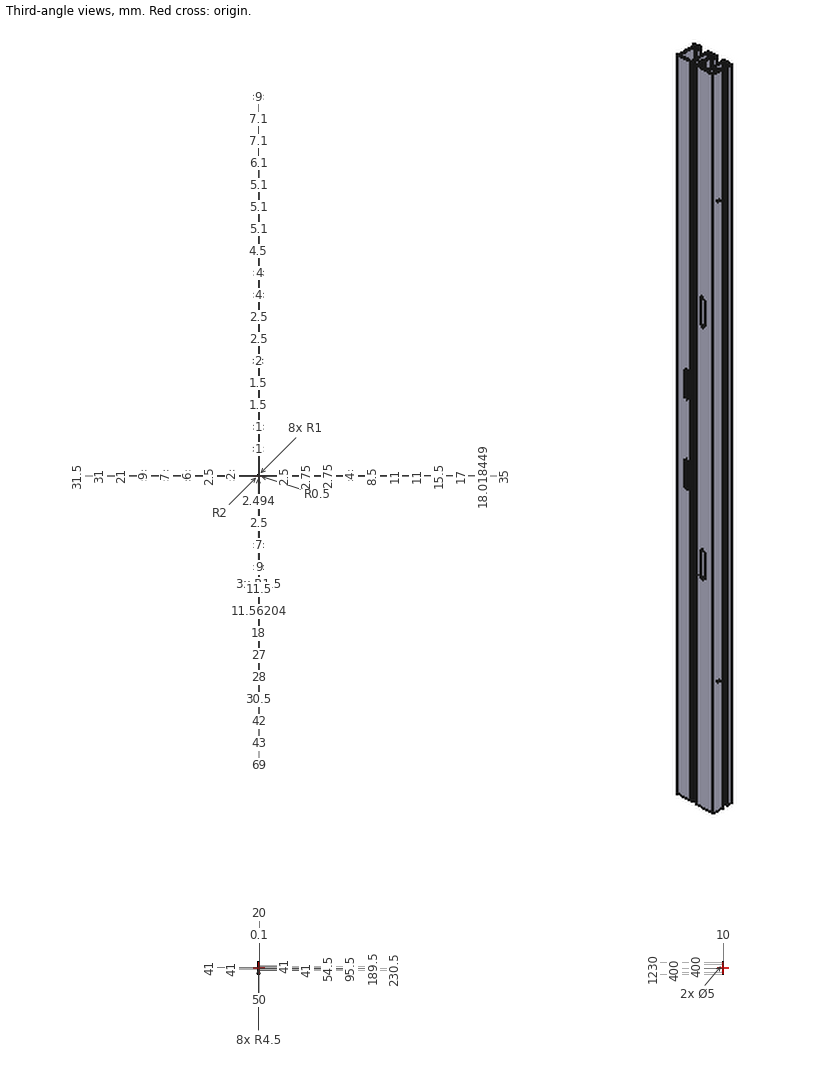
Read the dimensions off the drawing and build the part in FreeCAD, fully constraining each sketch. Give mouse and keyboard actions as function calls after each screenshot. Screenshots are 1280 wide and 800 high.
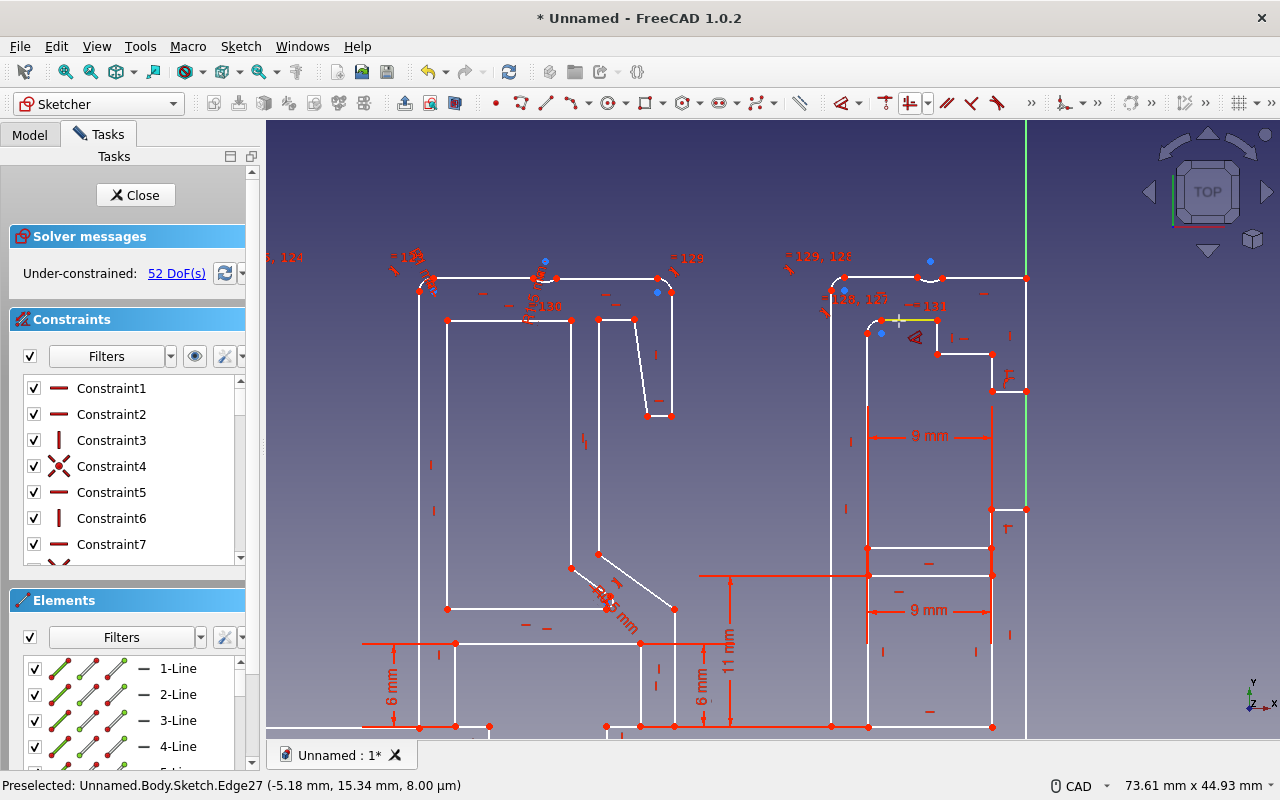
click(898, 320)
click(909, 354)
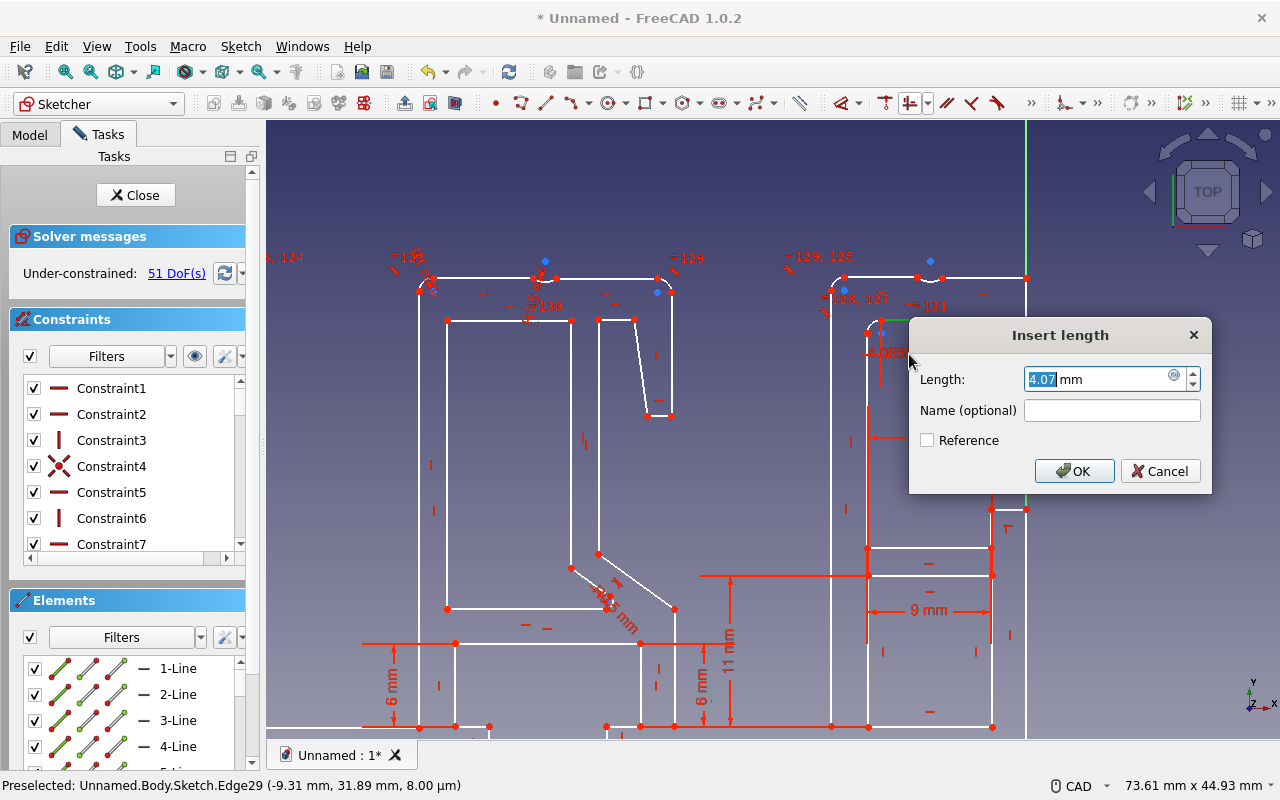
text(4)
key(Return)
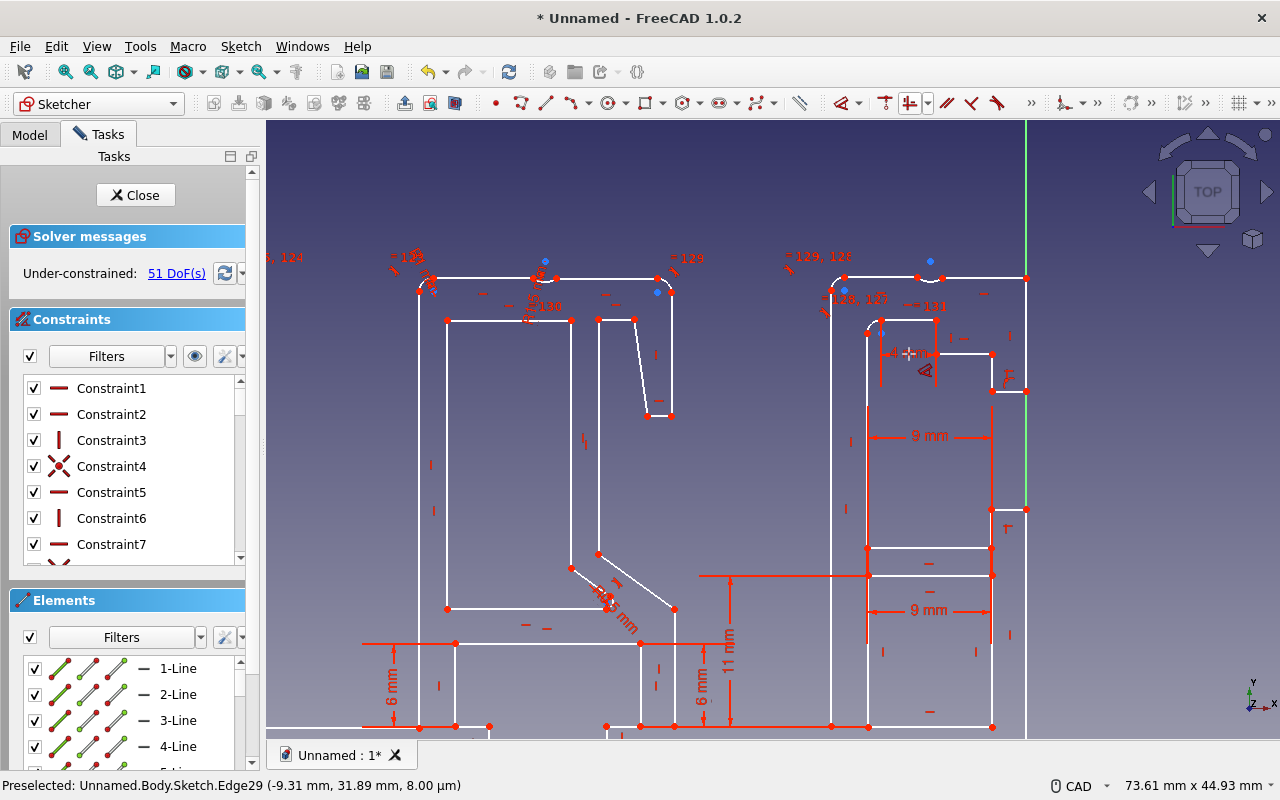
click(953, 354)
click(964, 320)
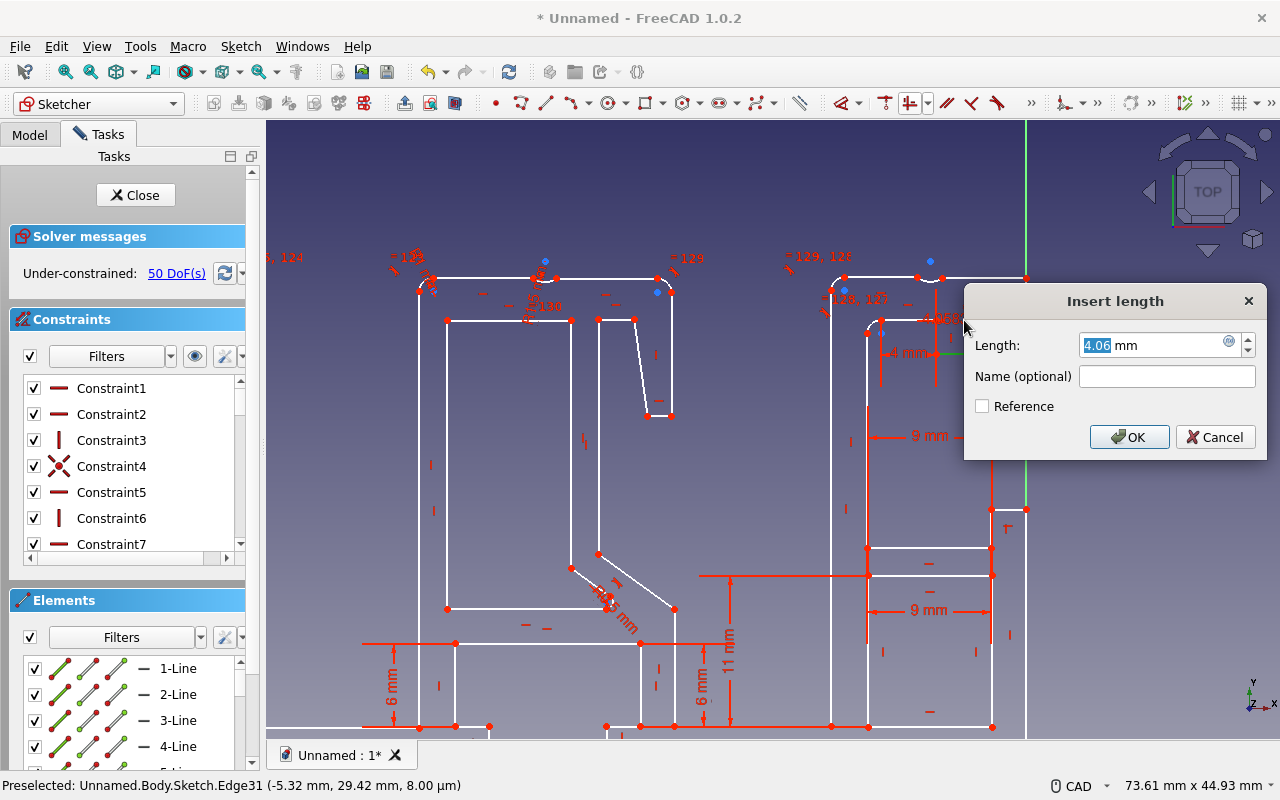
text(4)
key(Return)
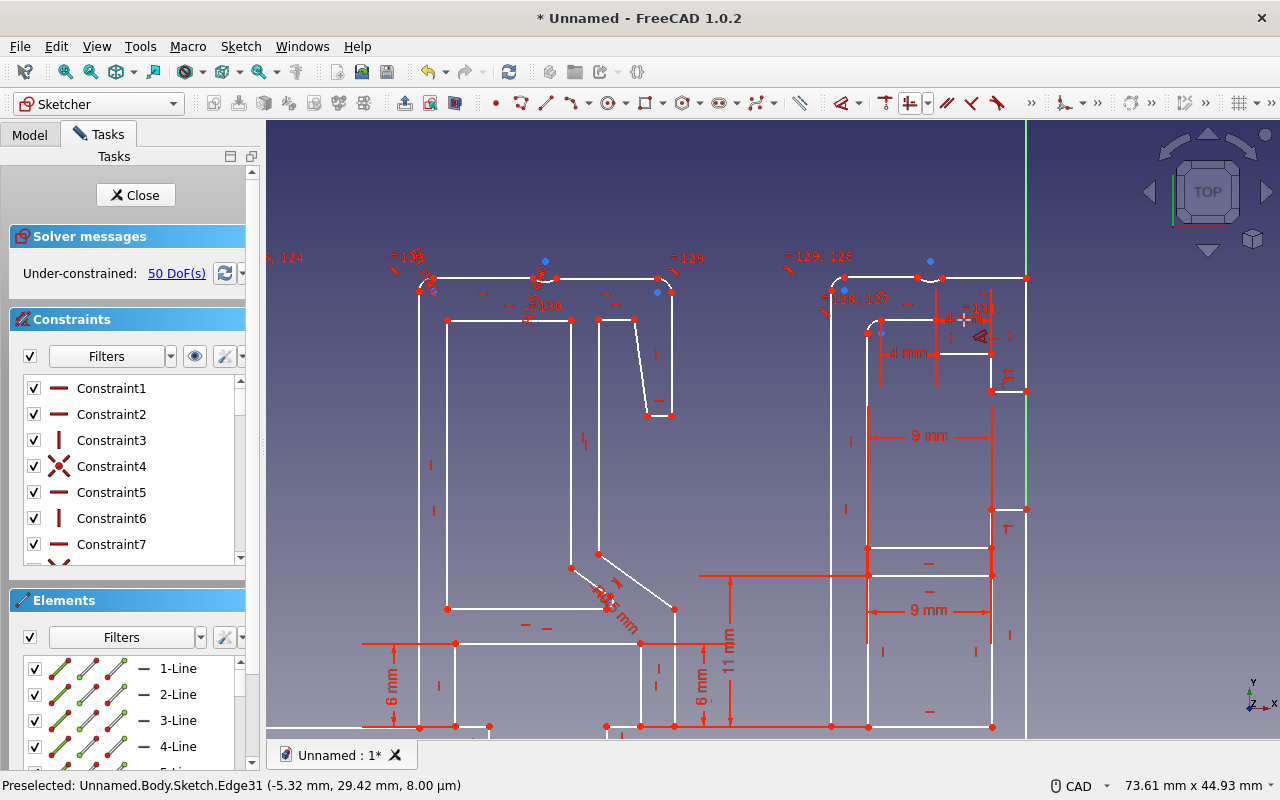
click(672, 379)
click(706, 355)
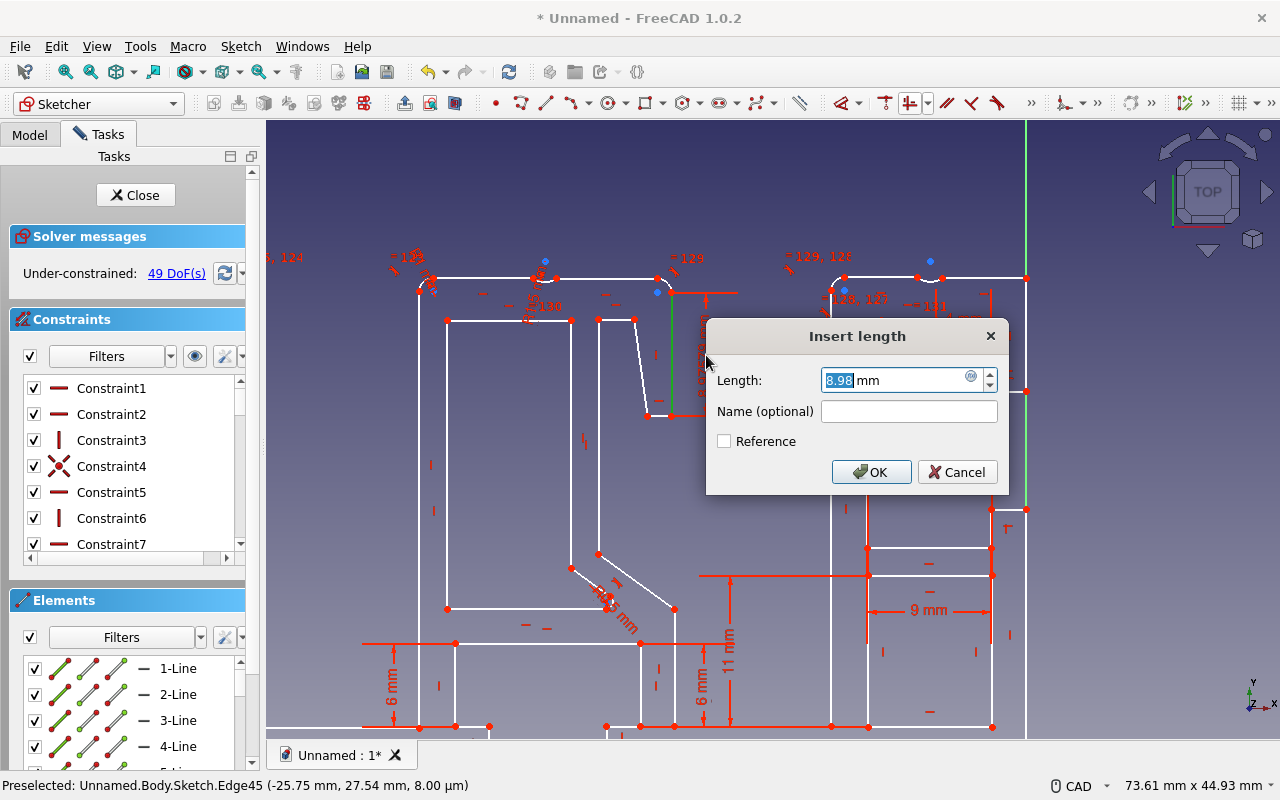
text(9)
key(Return)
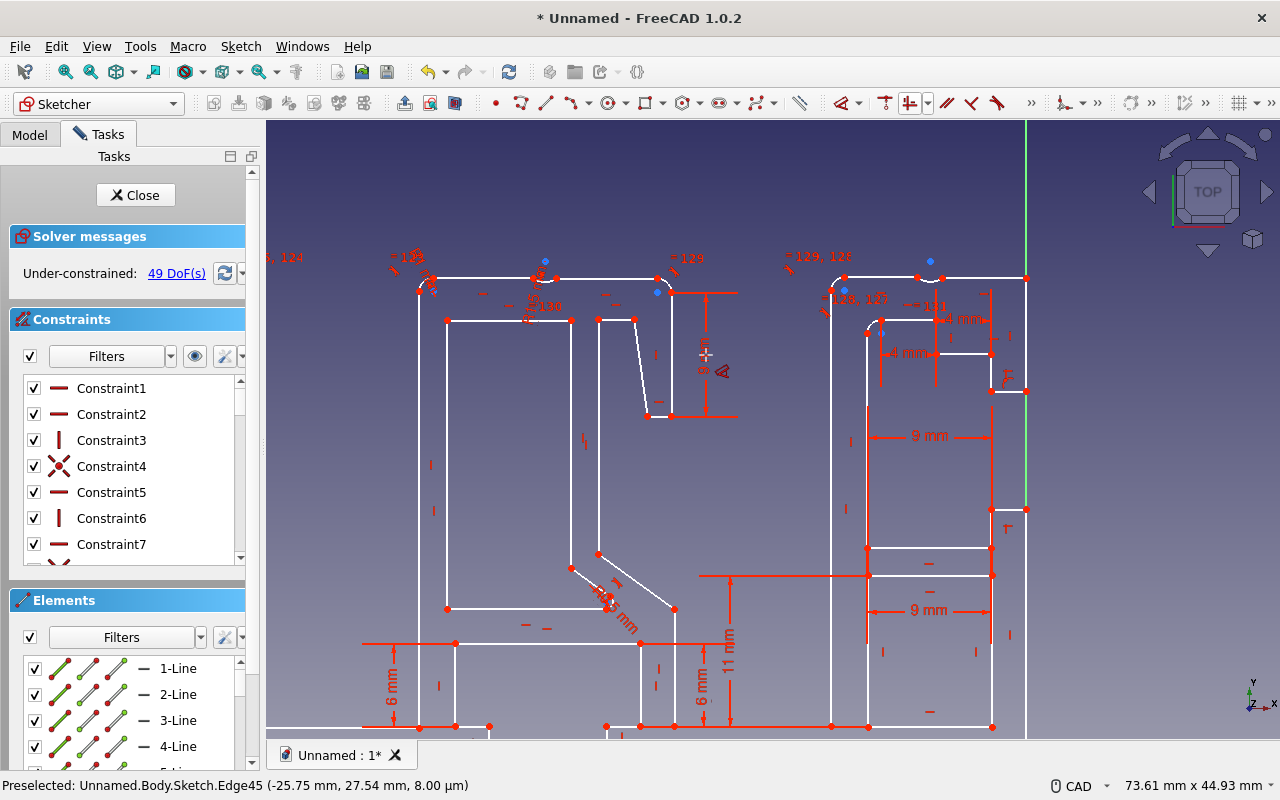
click(484, 321)
click(509, 355)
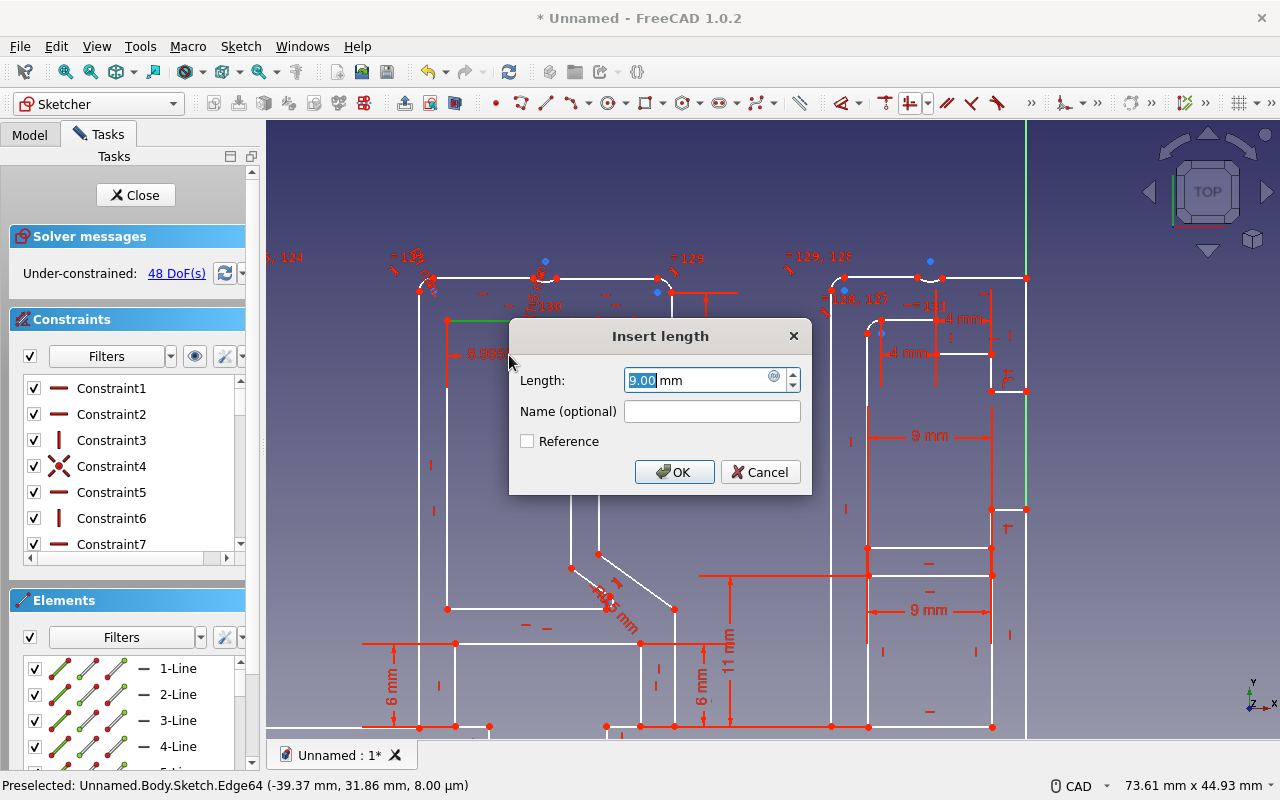
text(9)
key(Return)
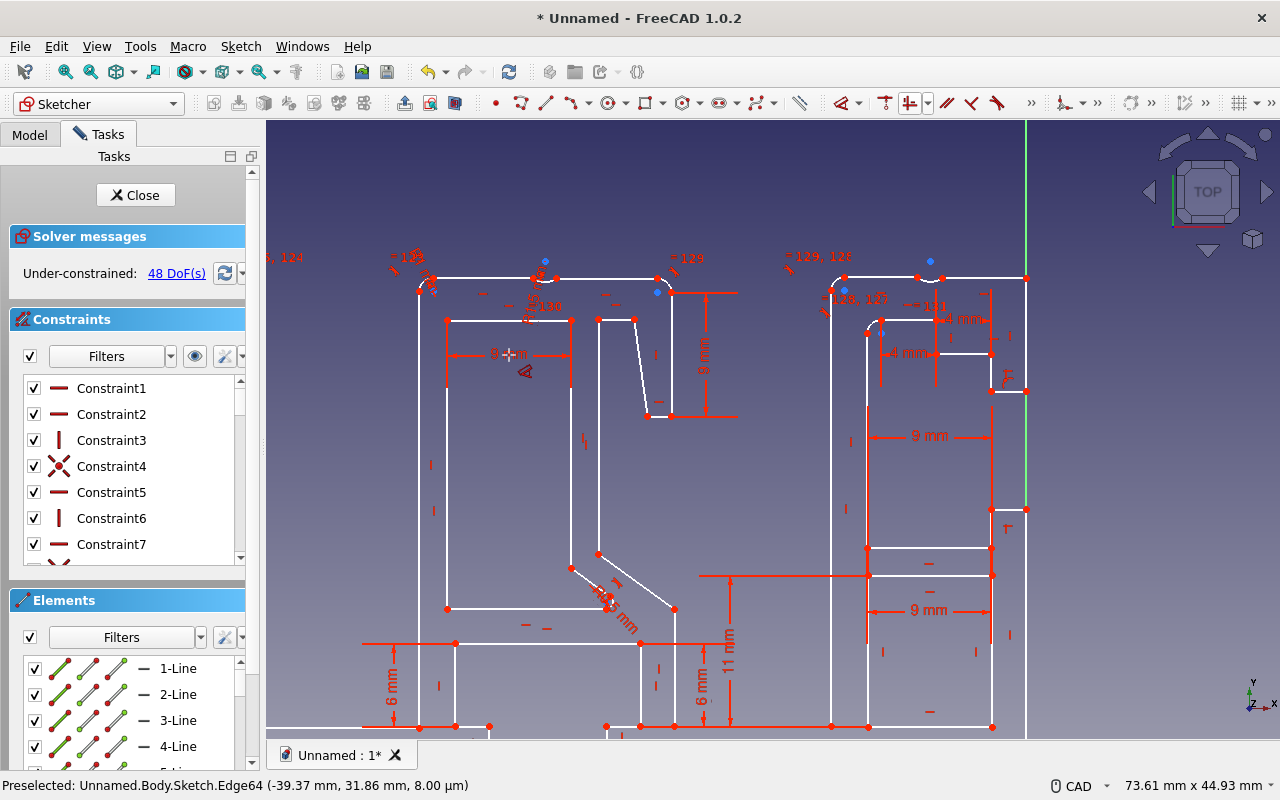
scroll(900, 321, down, 3)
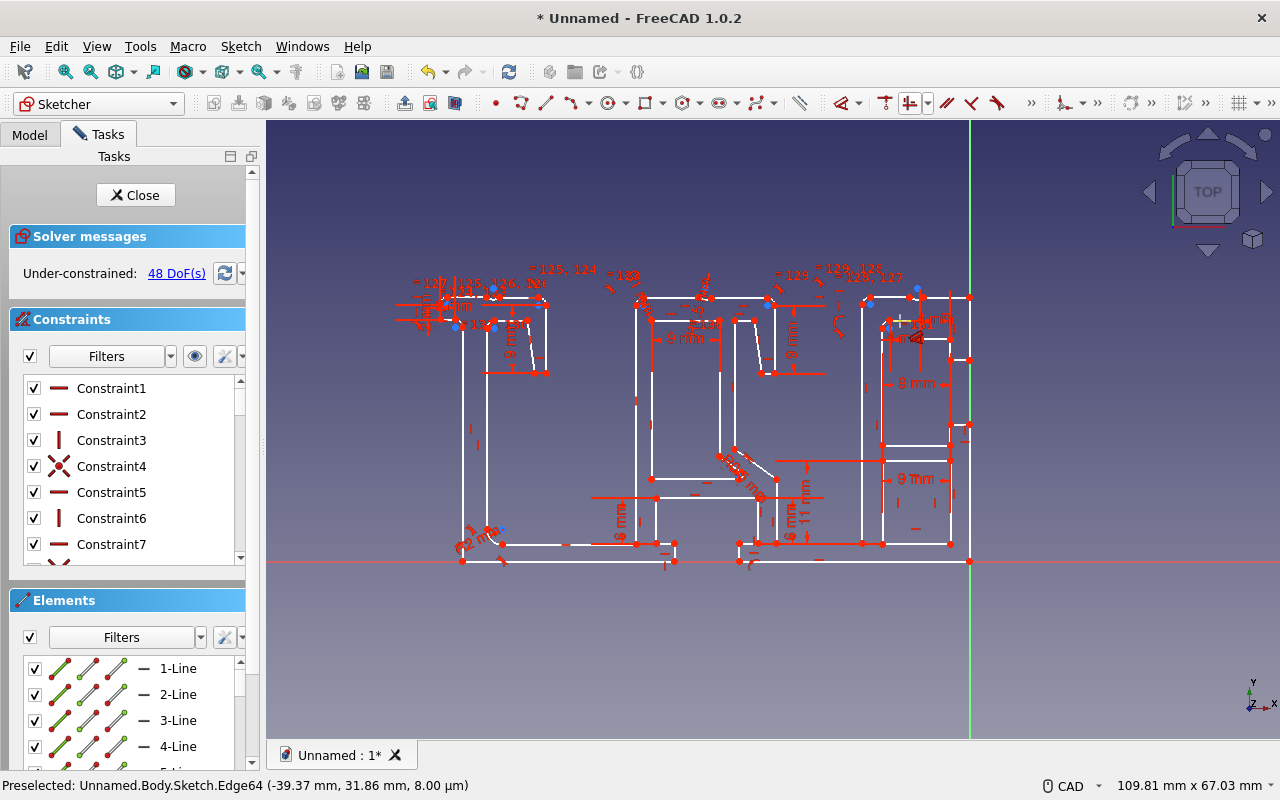
click(596, 545)
click(569, 579)